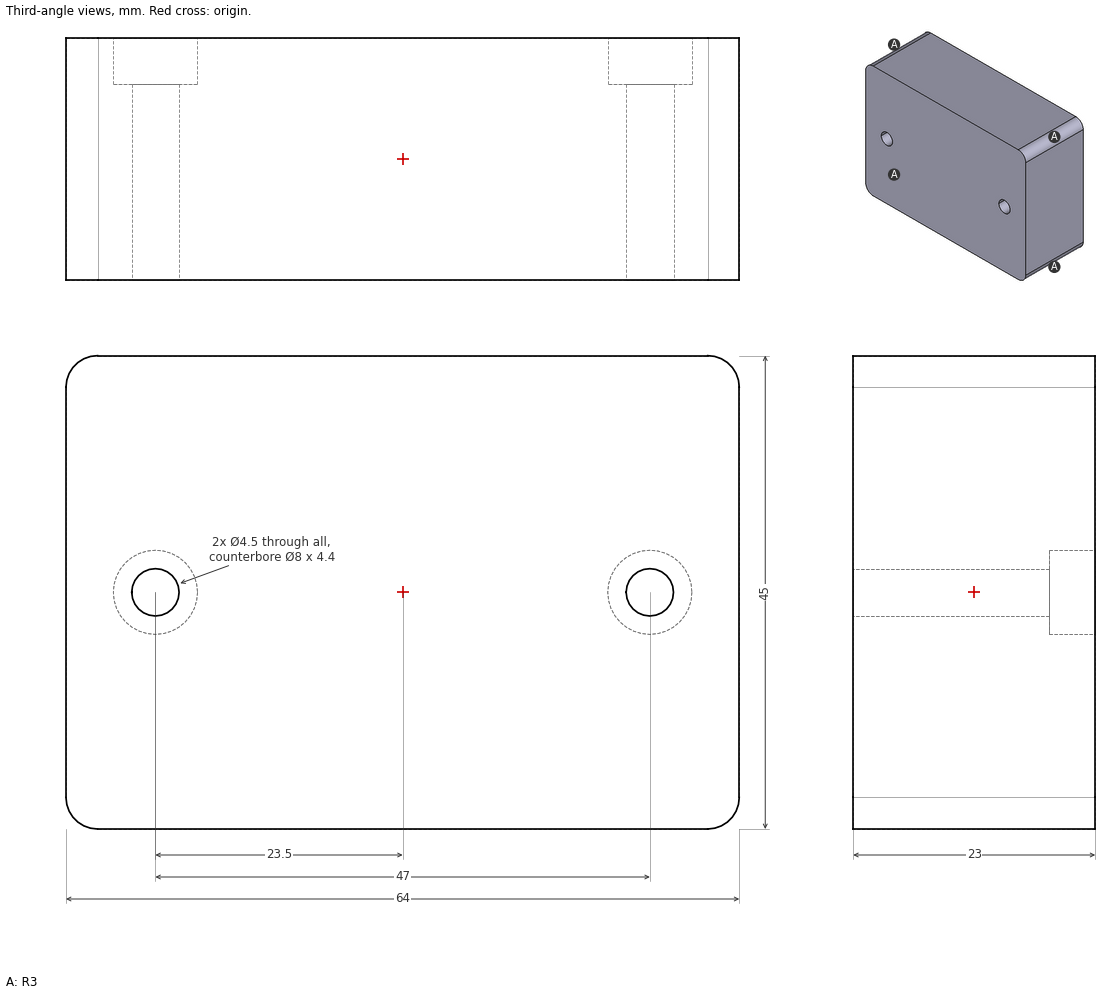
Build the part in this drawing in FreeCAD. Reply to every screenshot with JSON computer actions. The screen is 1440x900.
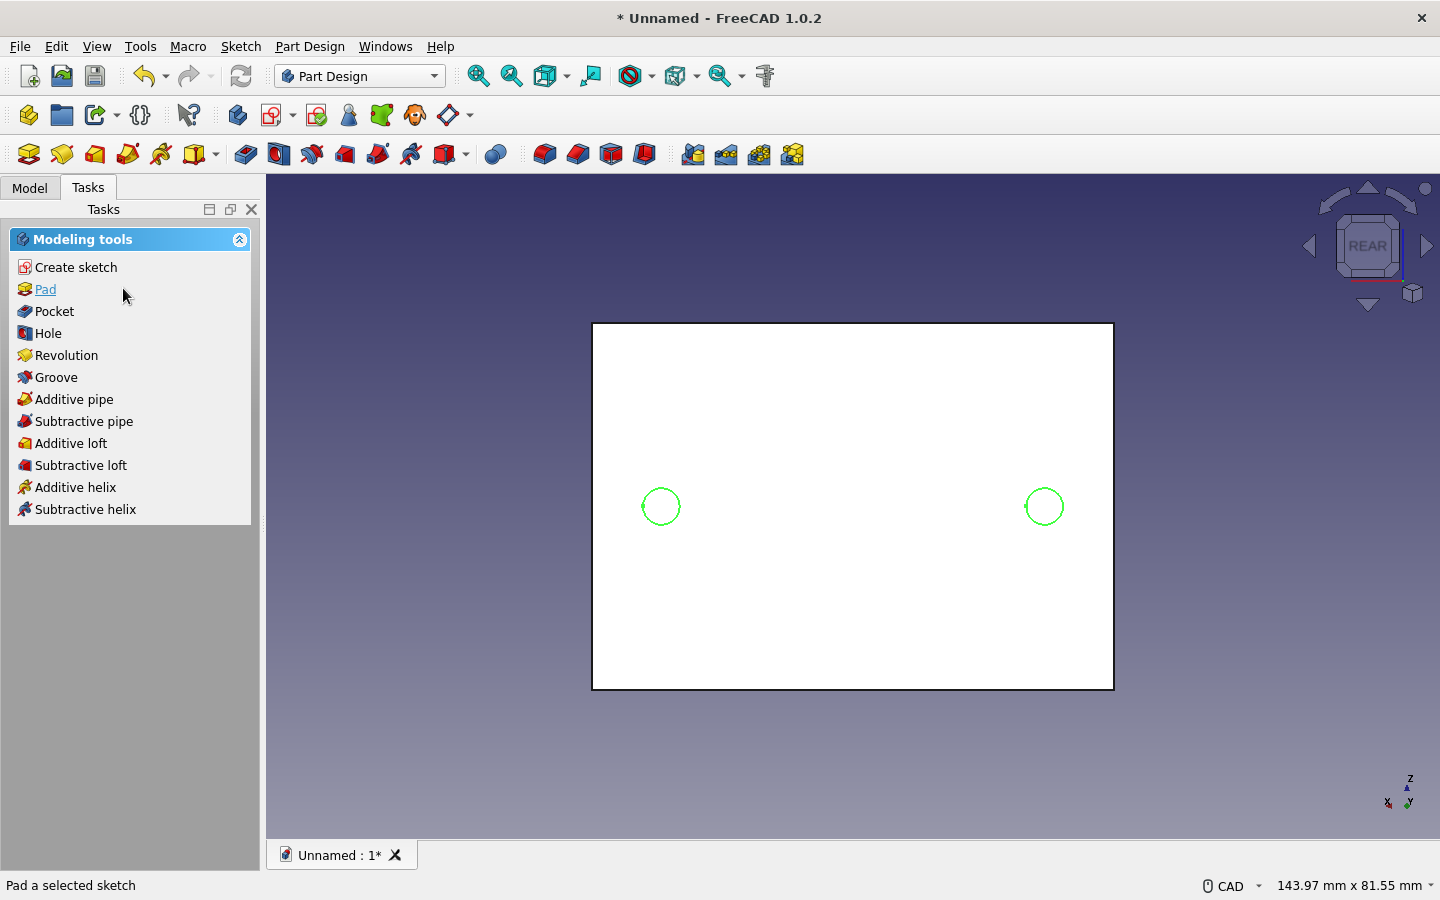
{"action": "left_click", "coordinate": [279, 154]}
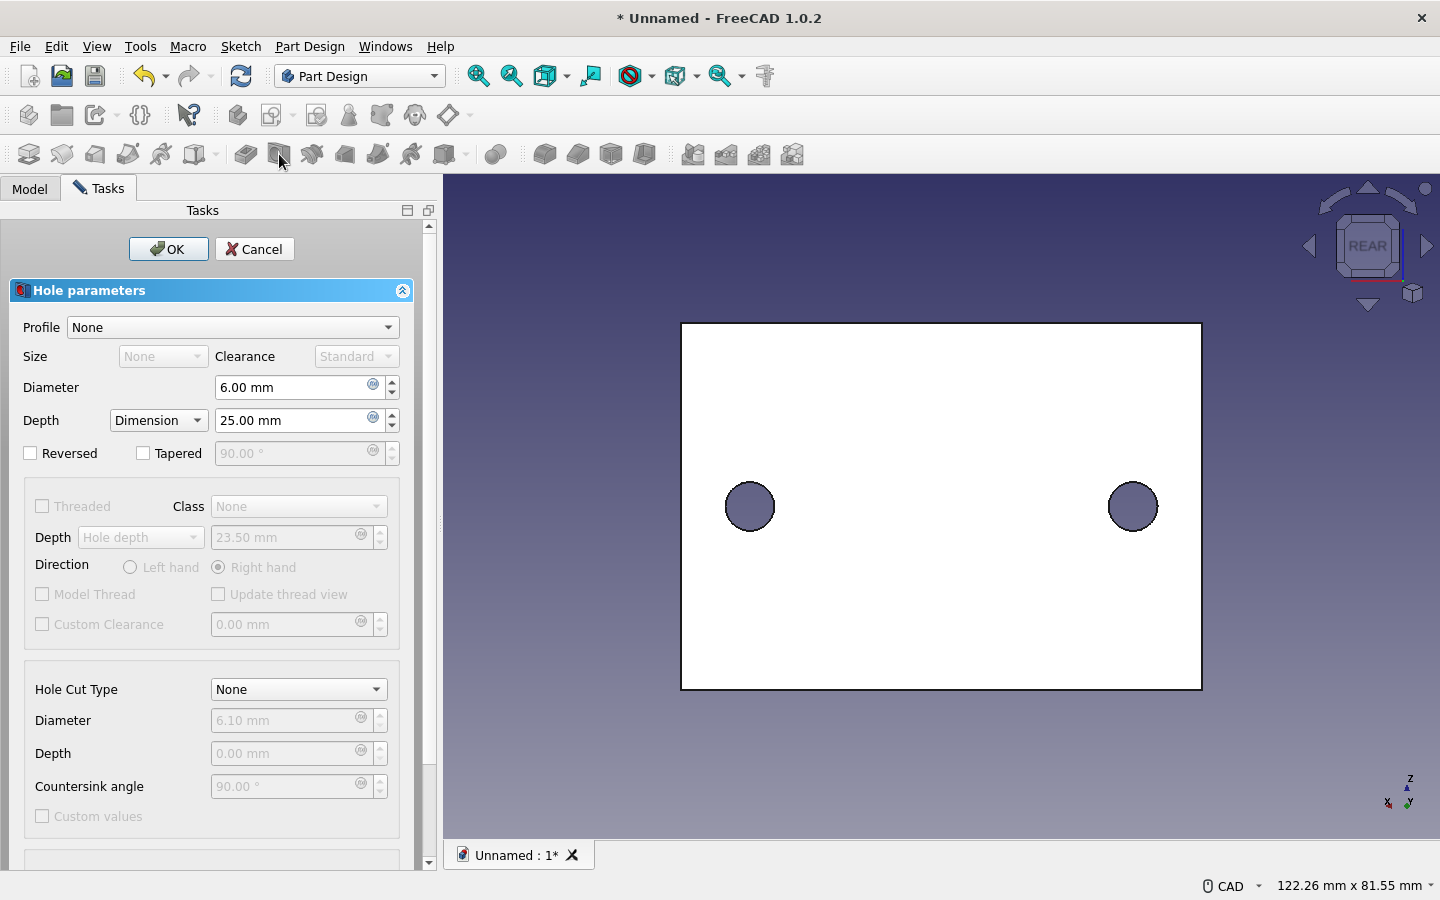
{"action": "triple_click", "coordinate": [300, 388]}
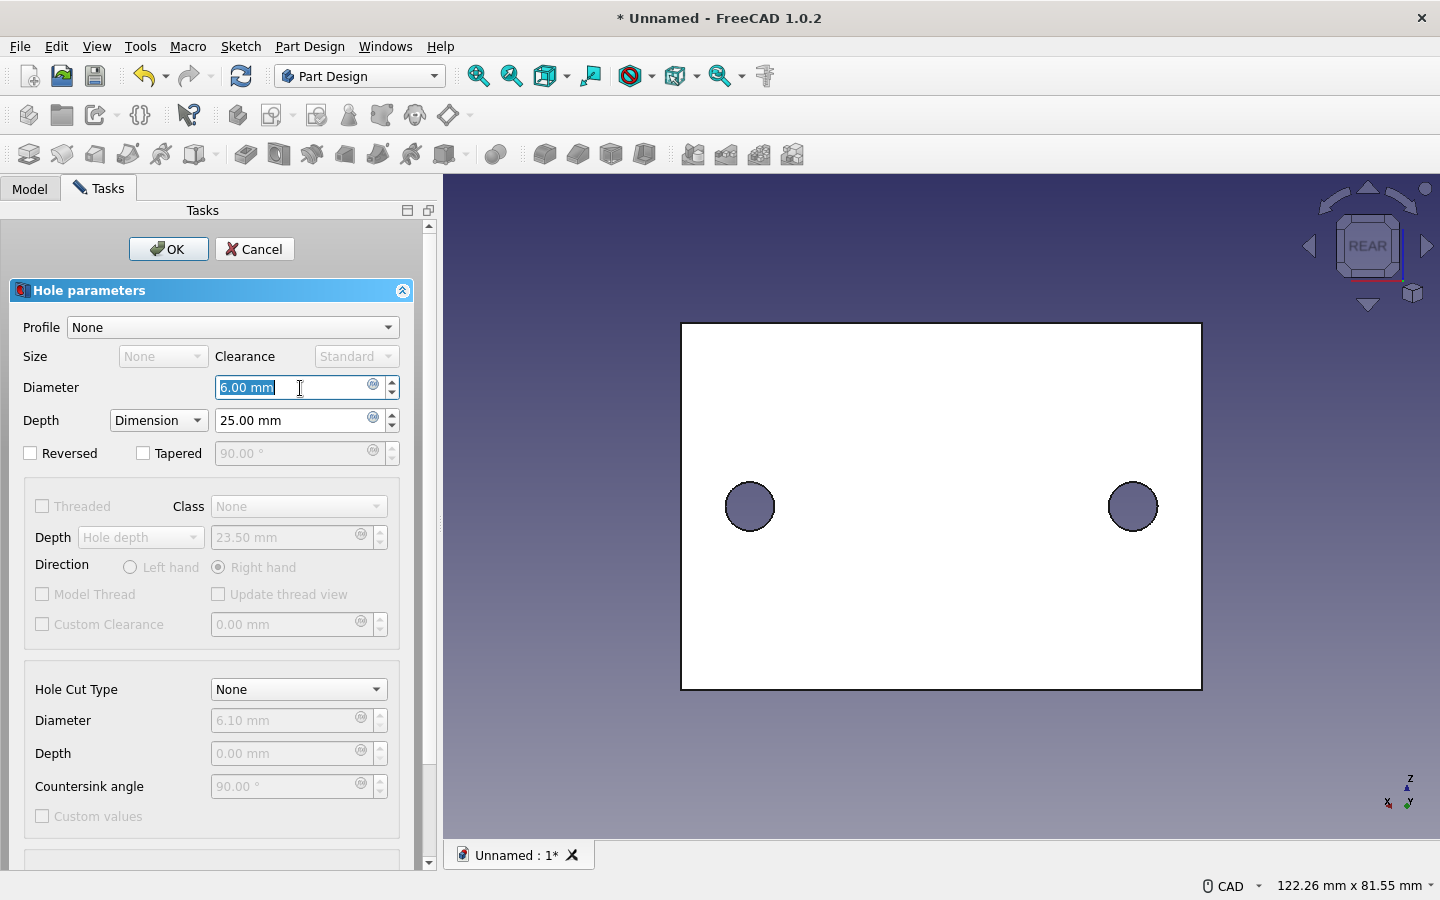
{"action": "type", "text": "4.5"}
{"action": "key", "text": "Tab"}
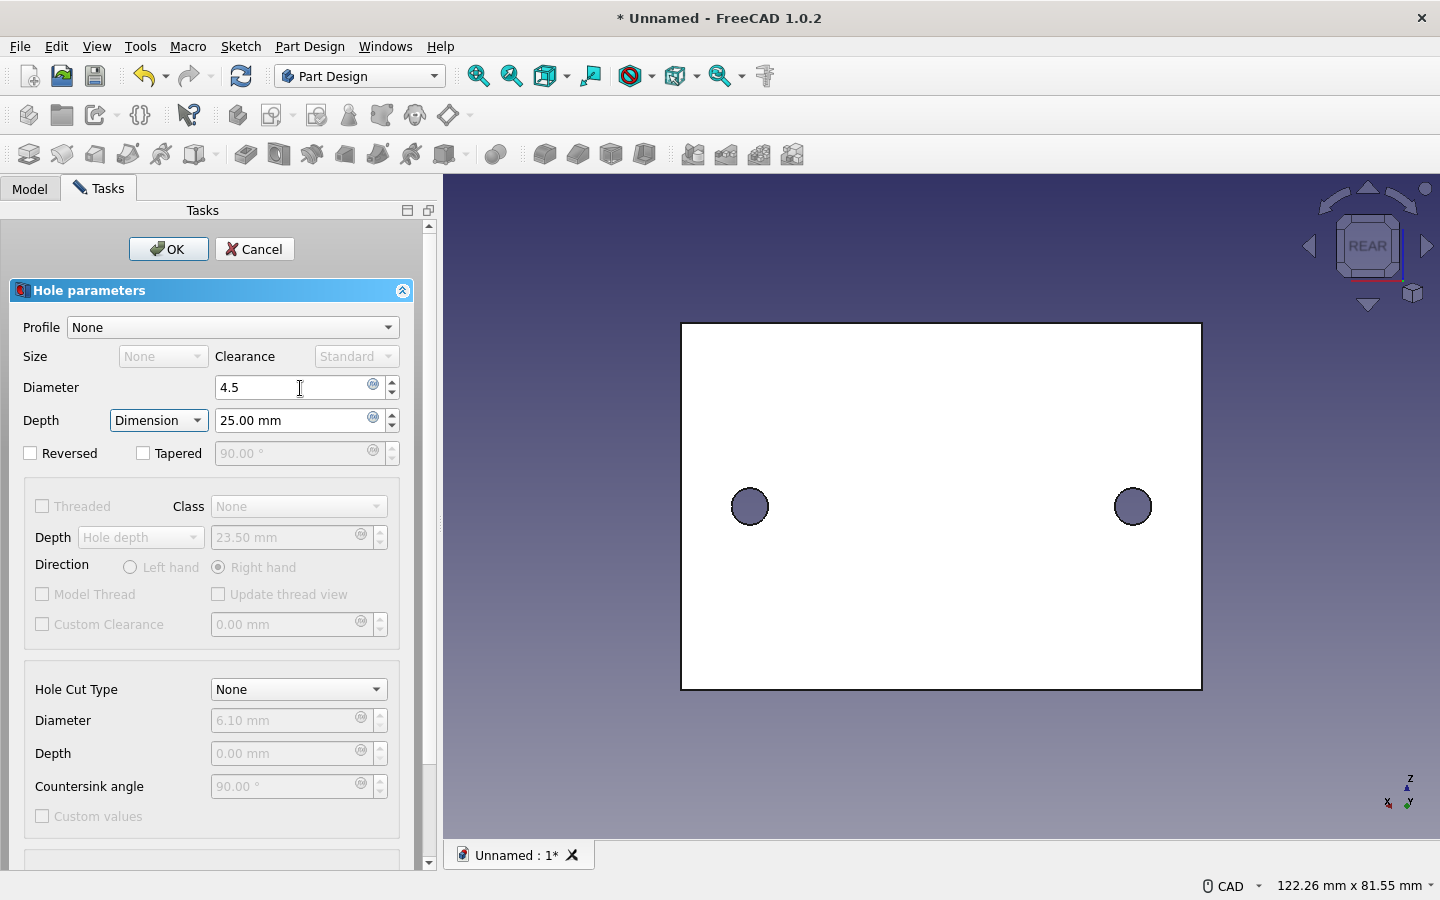
{"action": "left_click", "coordinate": [160, 420]}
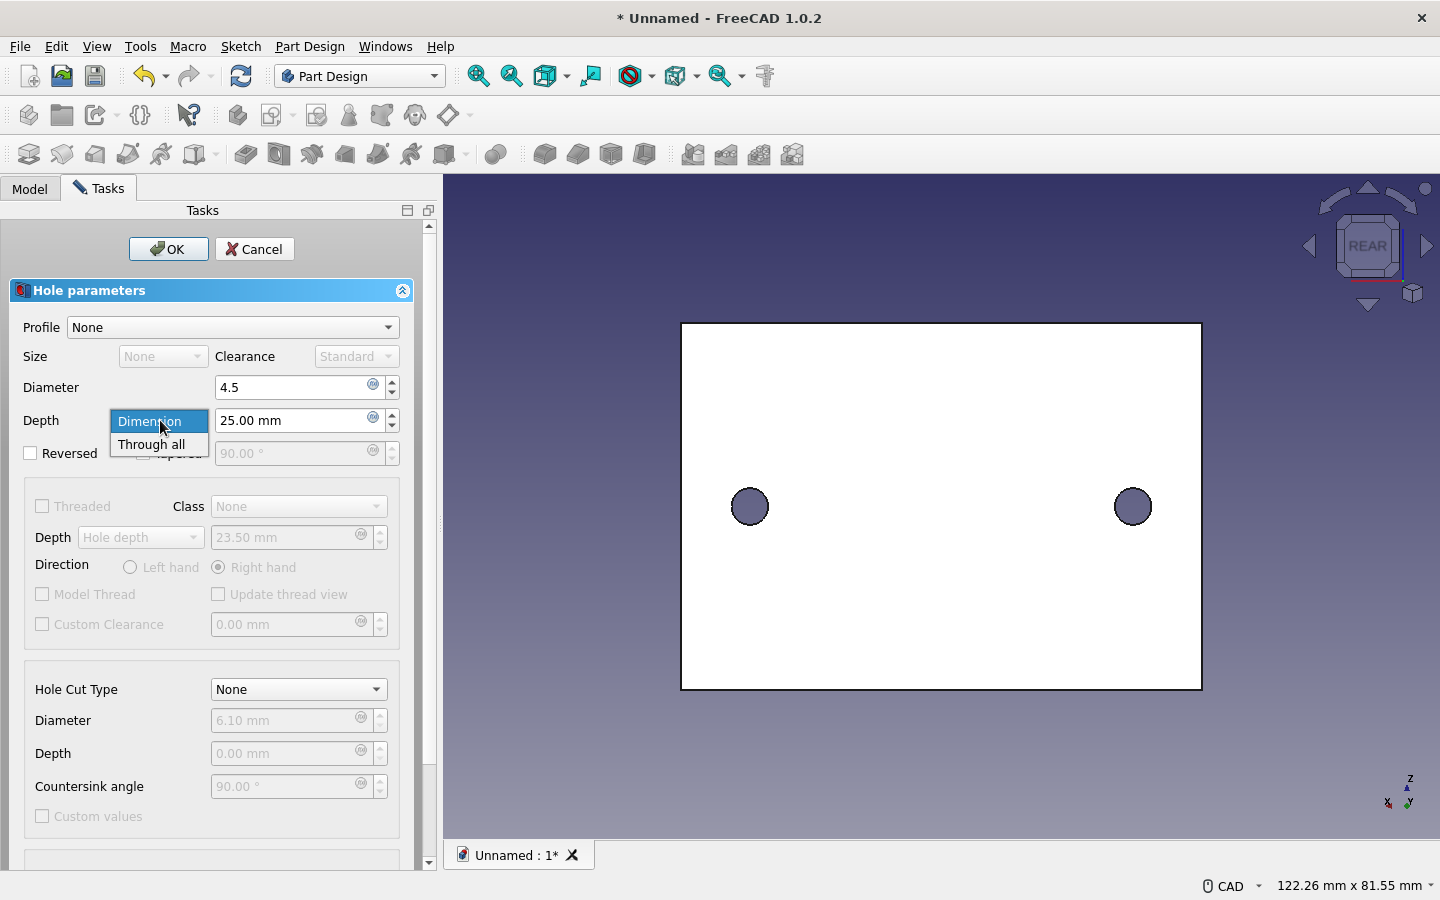
{"action": "left_click", "coordinate": [158, 444]}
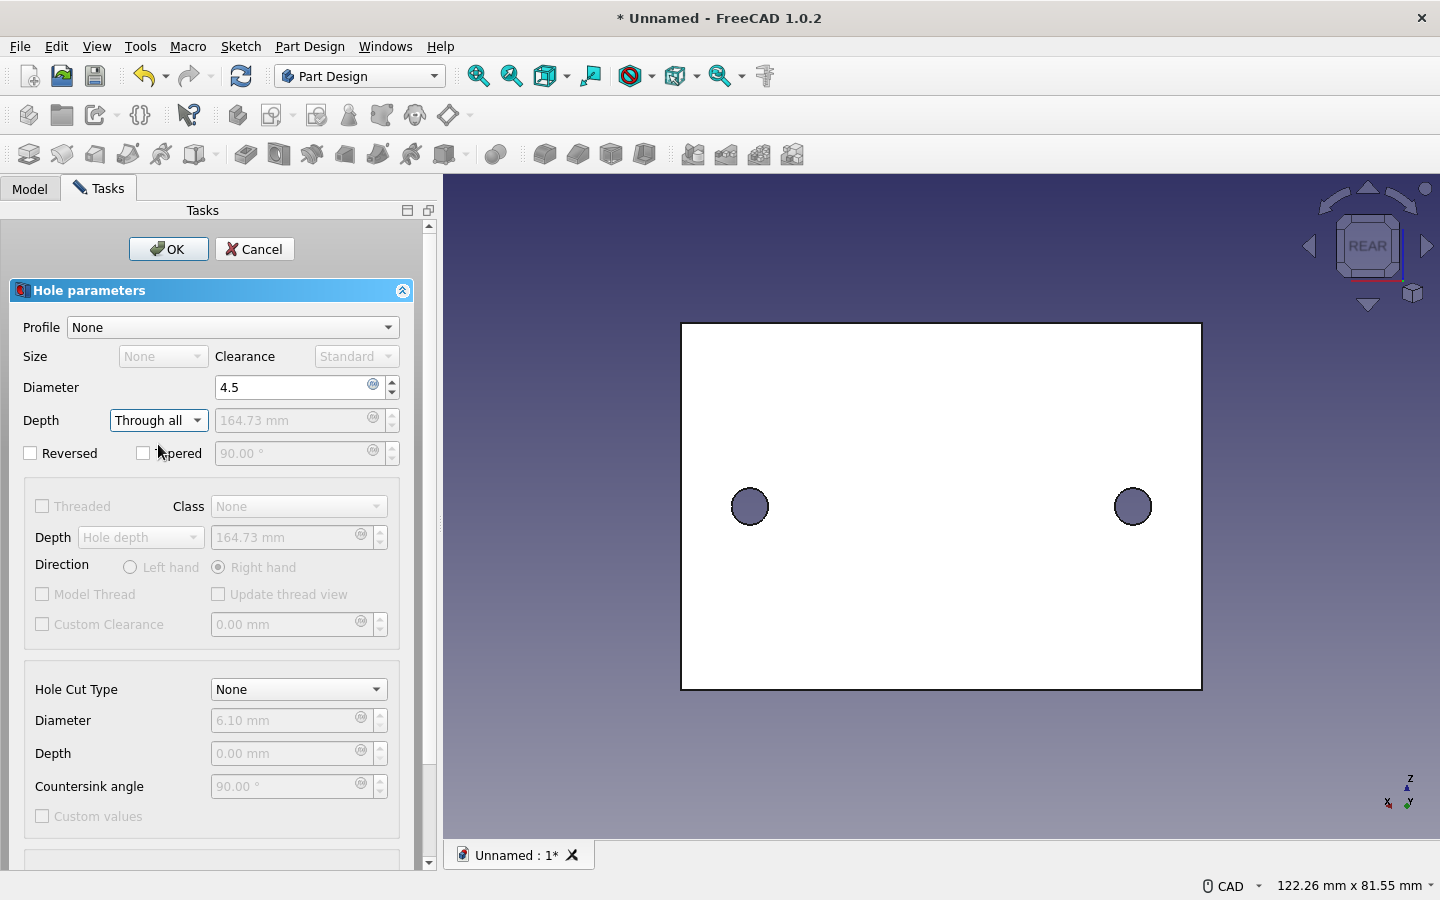
{"action": "left_click", "coordinate": [300, 690]}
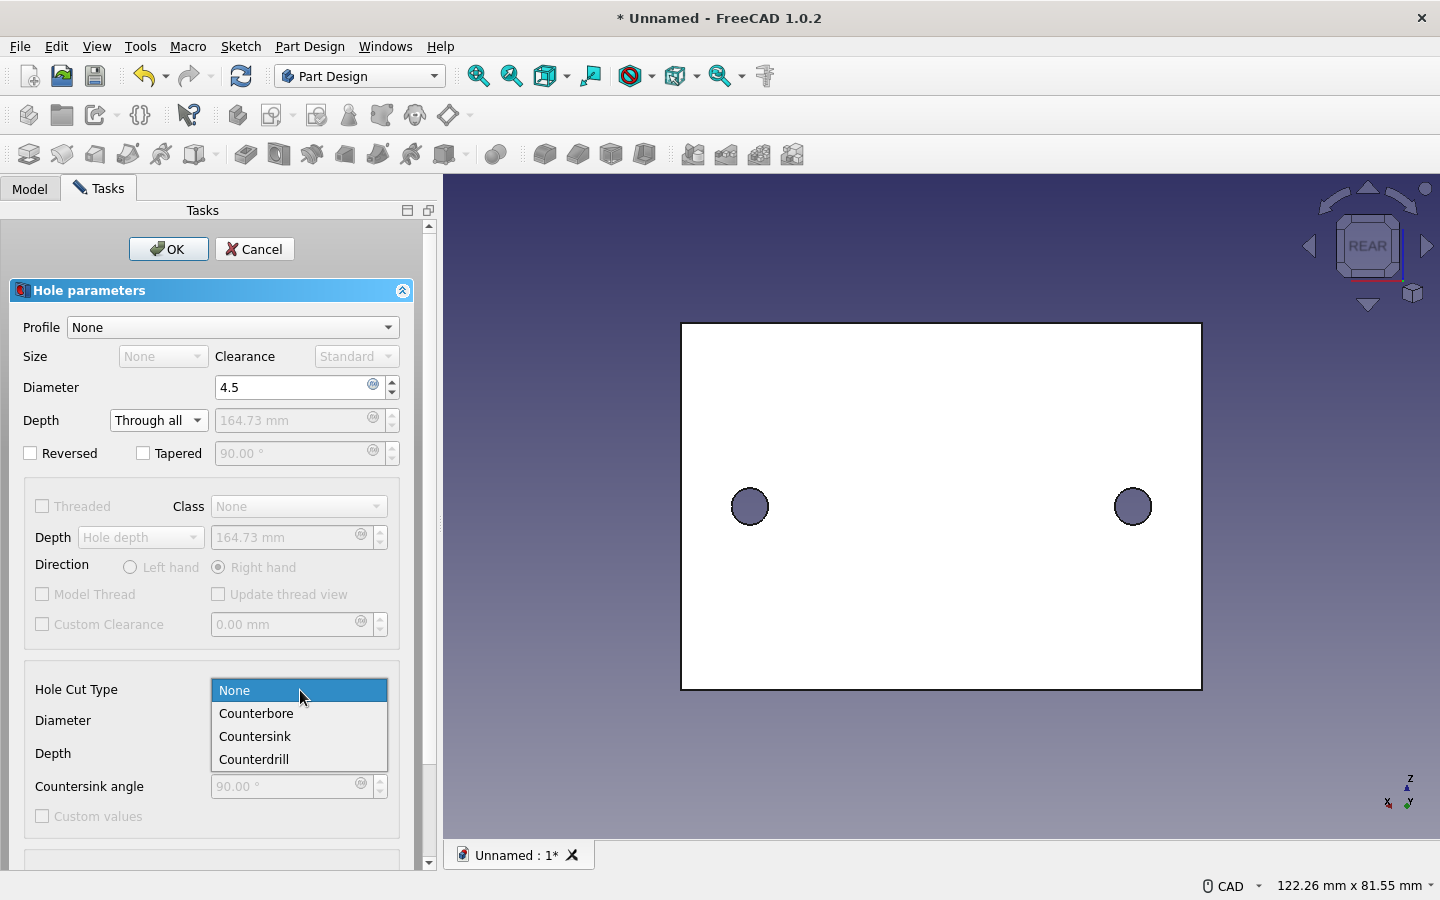
{"action": "left_click", "coordinate": [298, 714]}